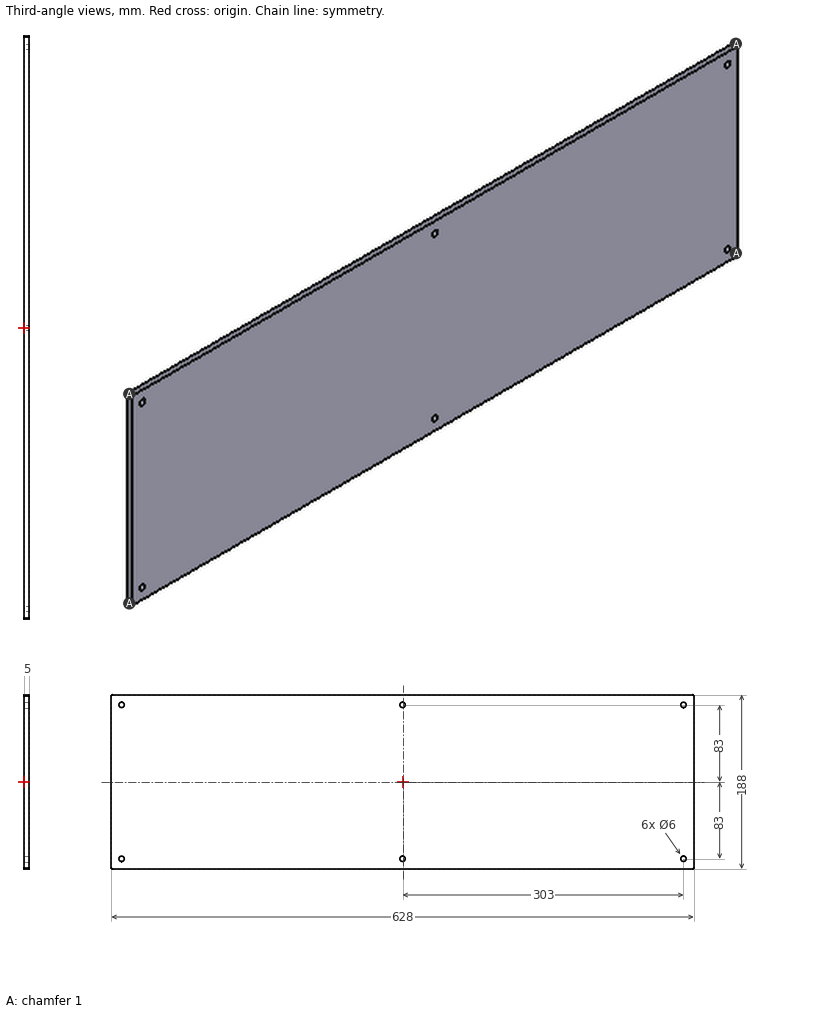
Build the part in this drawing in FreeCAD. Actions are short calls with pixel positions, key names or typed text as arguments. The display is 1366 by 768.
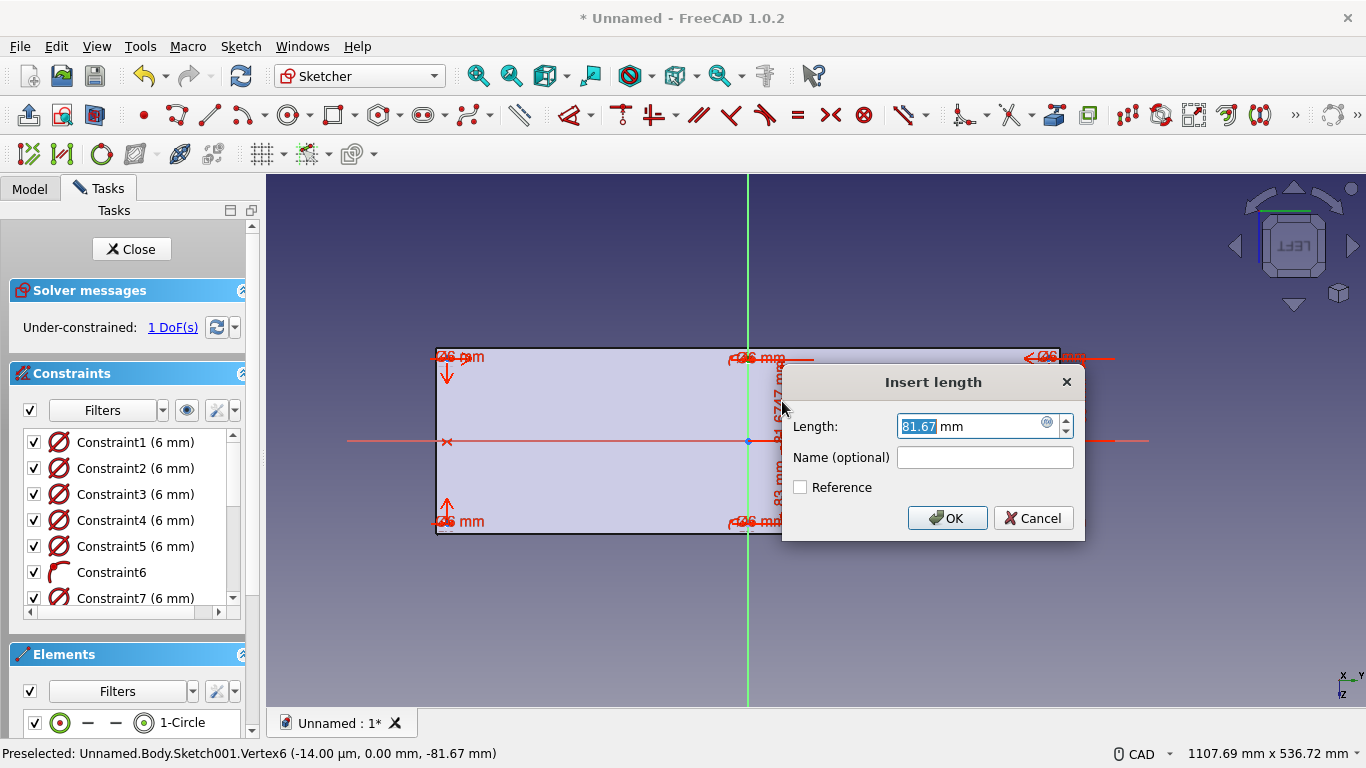
text(83)
key(Return)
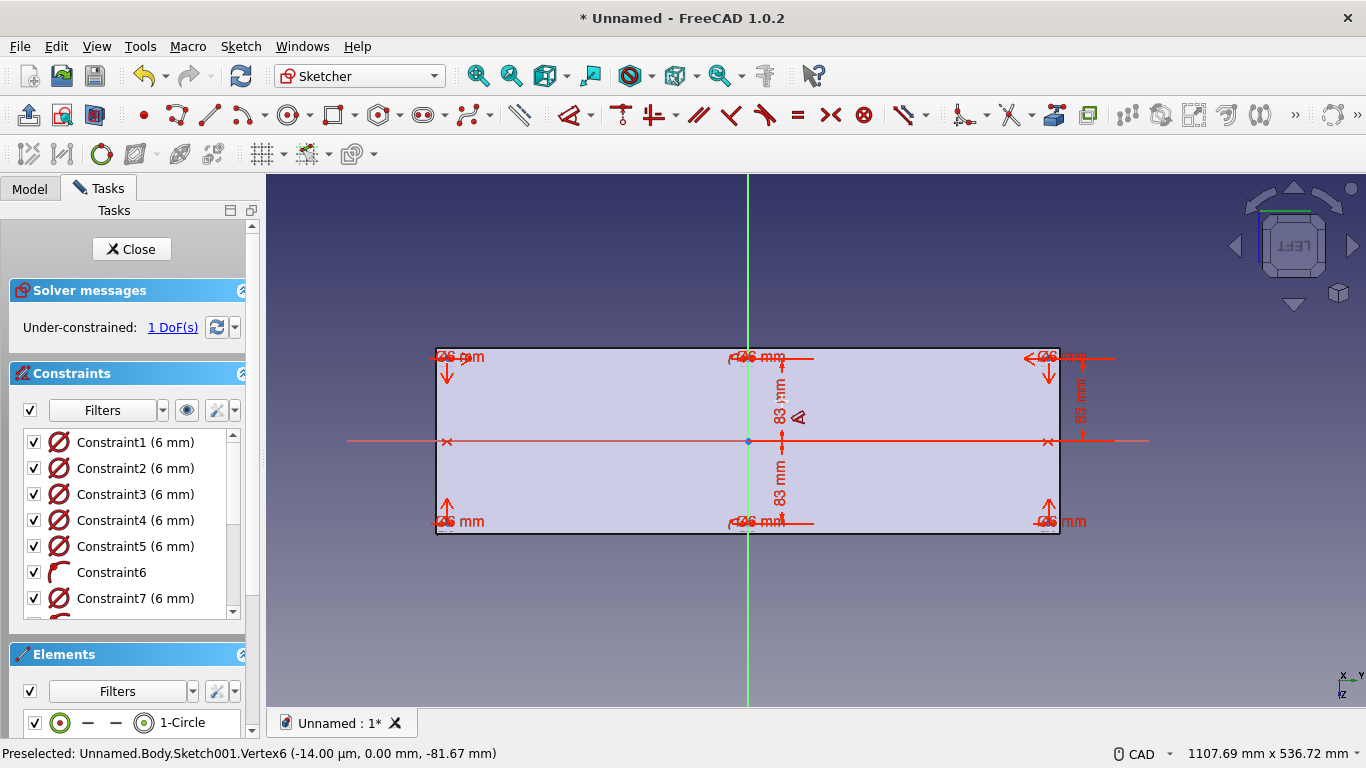
click(1049, 359)
click(899, 325)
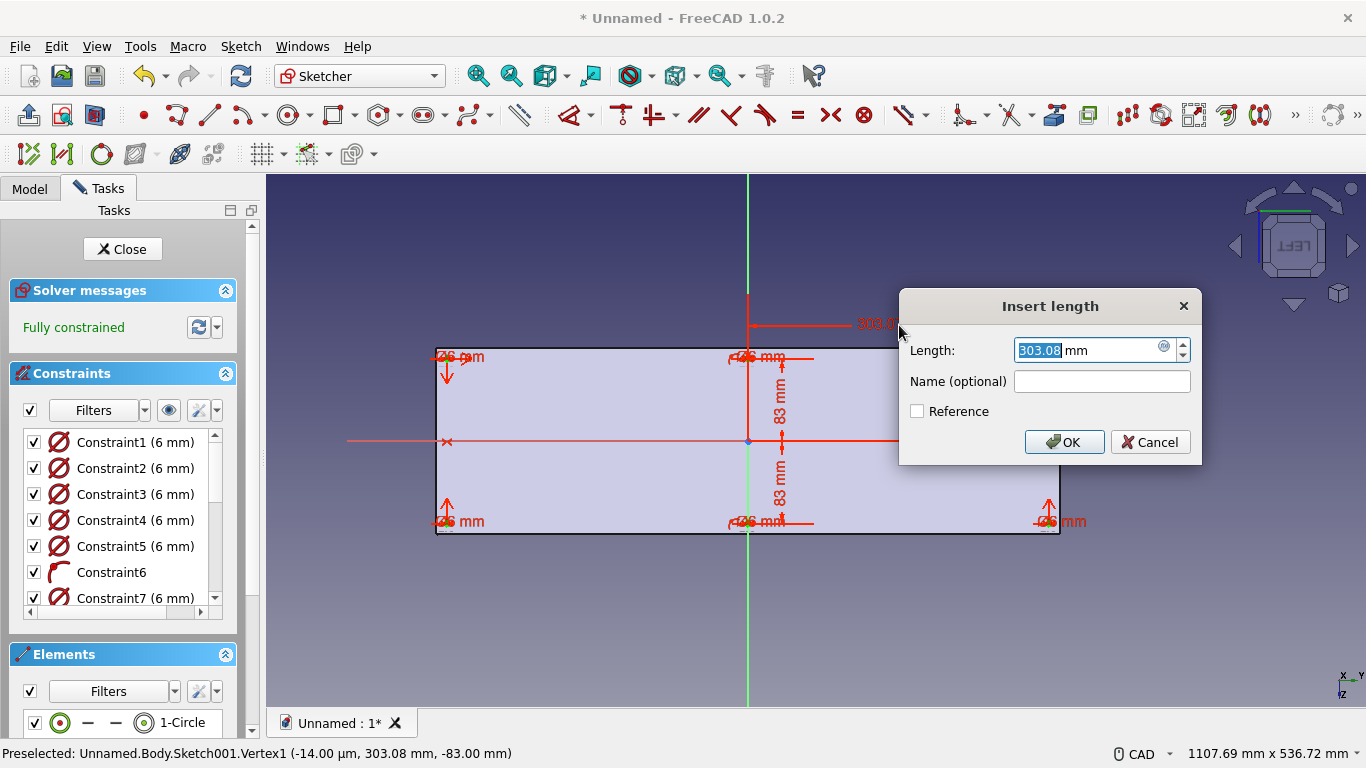
text(303)
key(Return)
key(Escape)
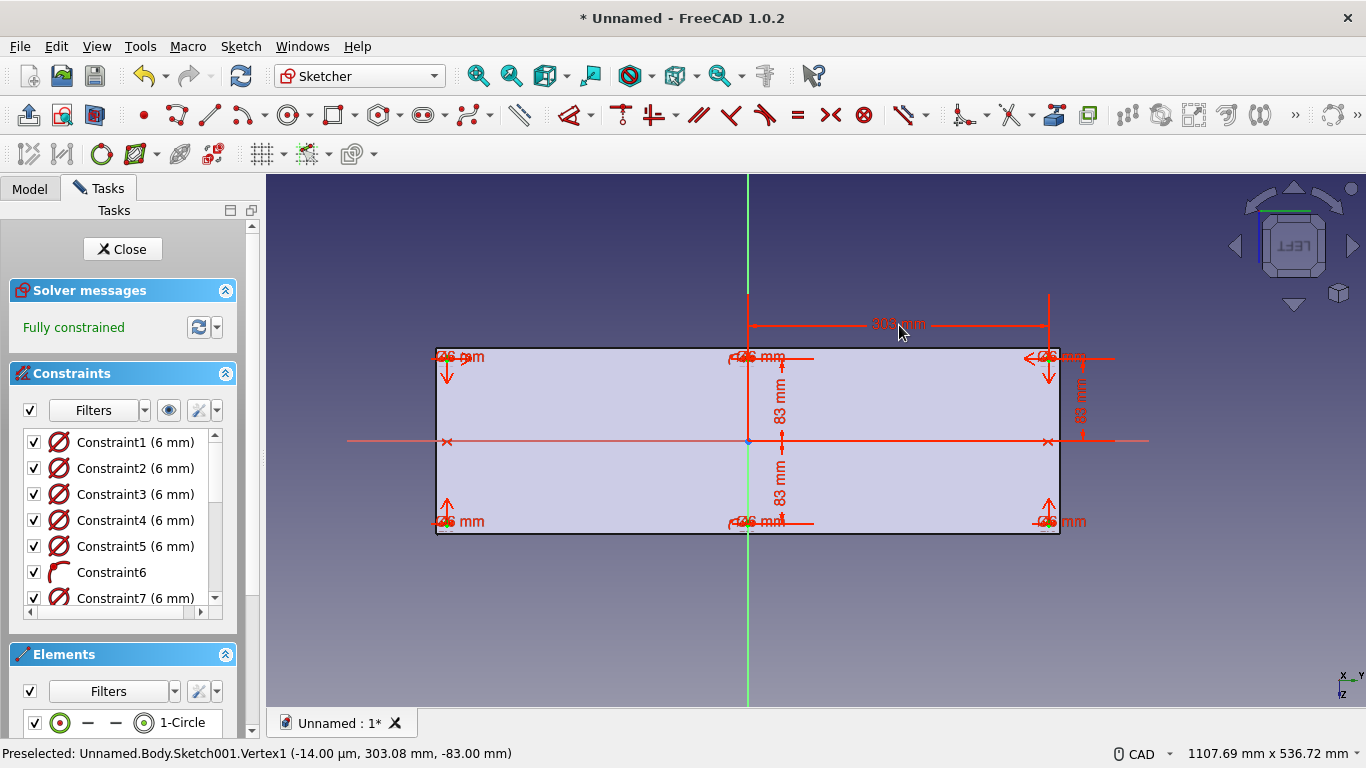
click(123, 249)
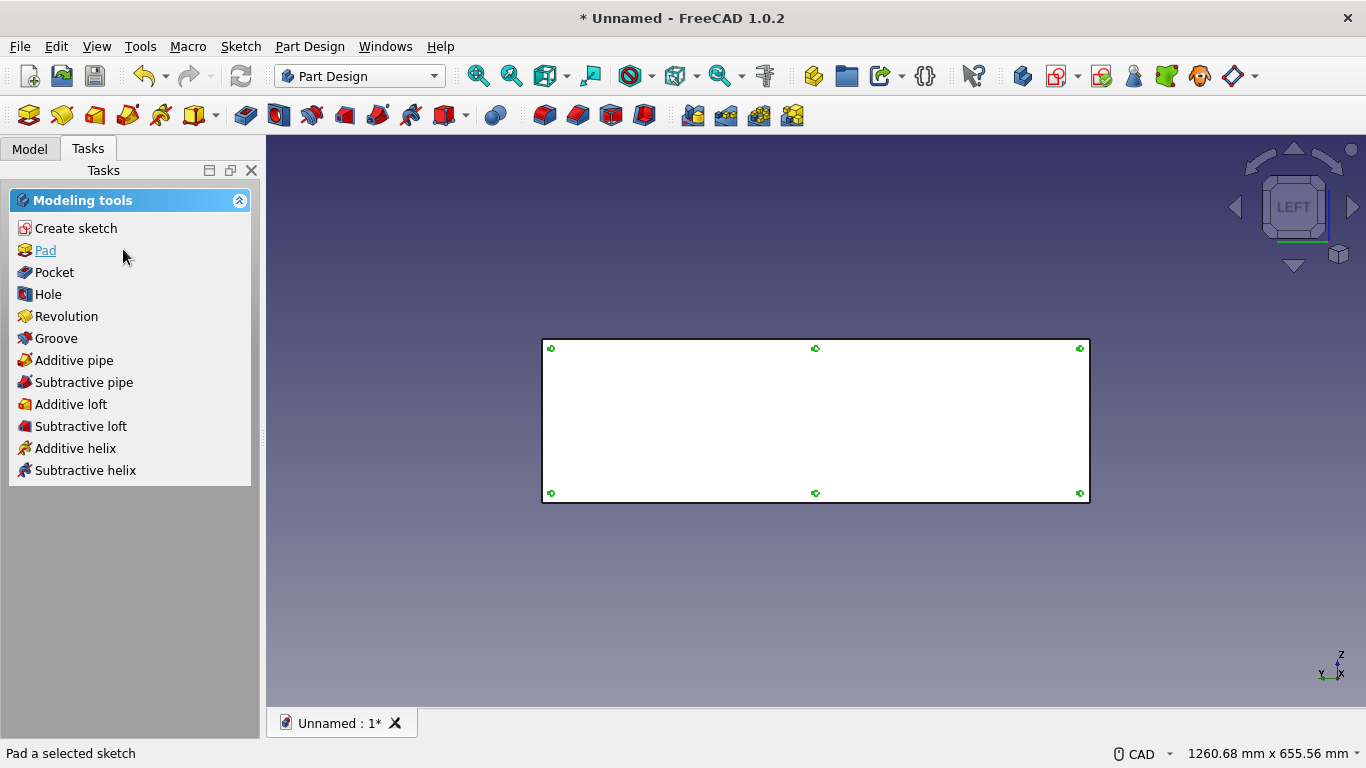
click(246, 116)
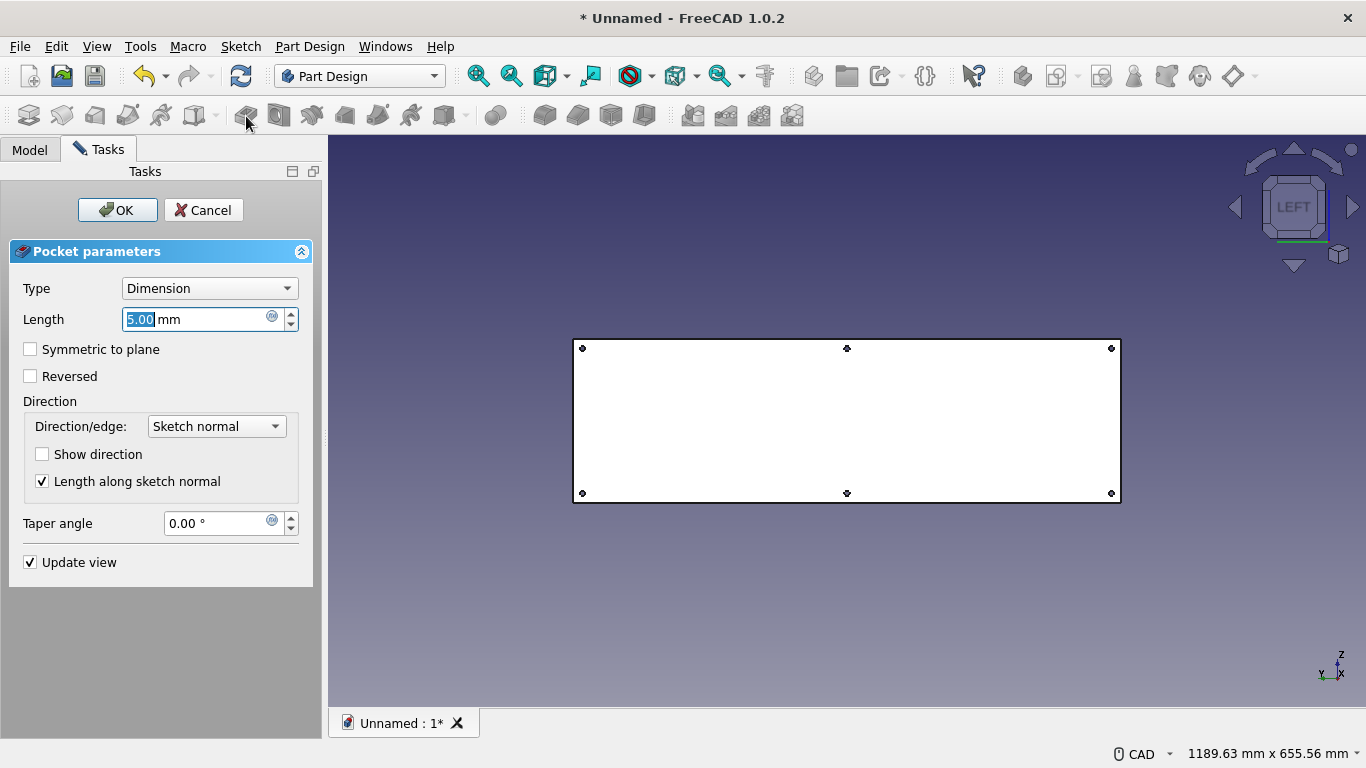
click(210, 288)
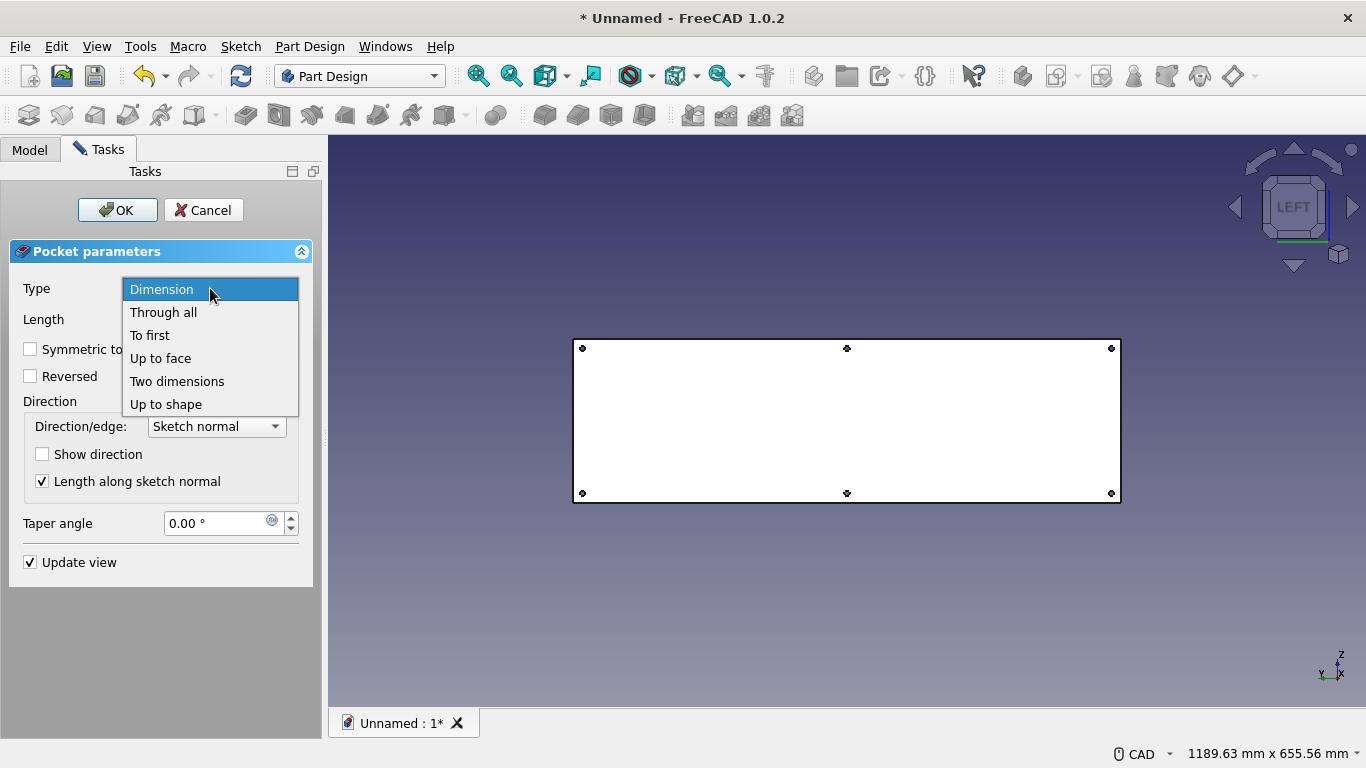
click(208, 312)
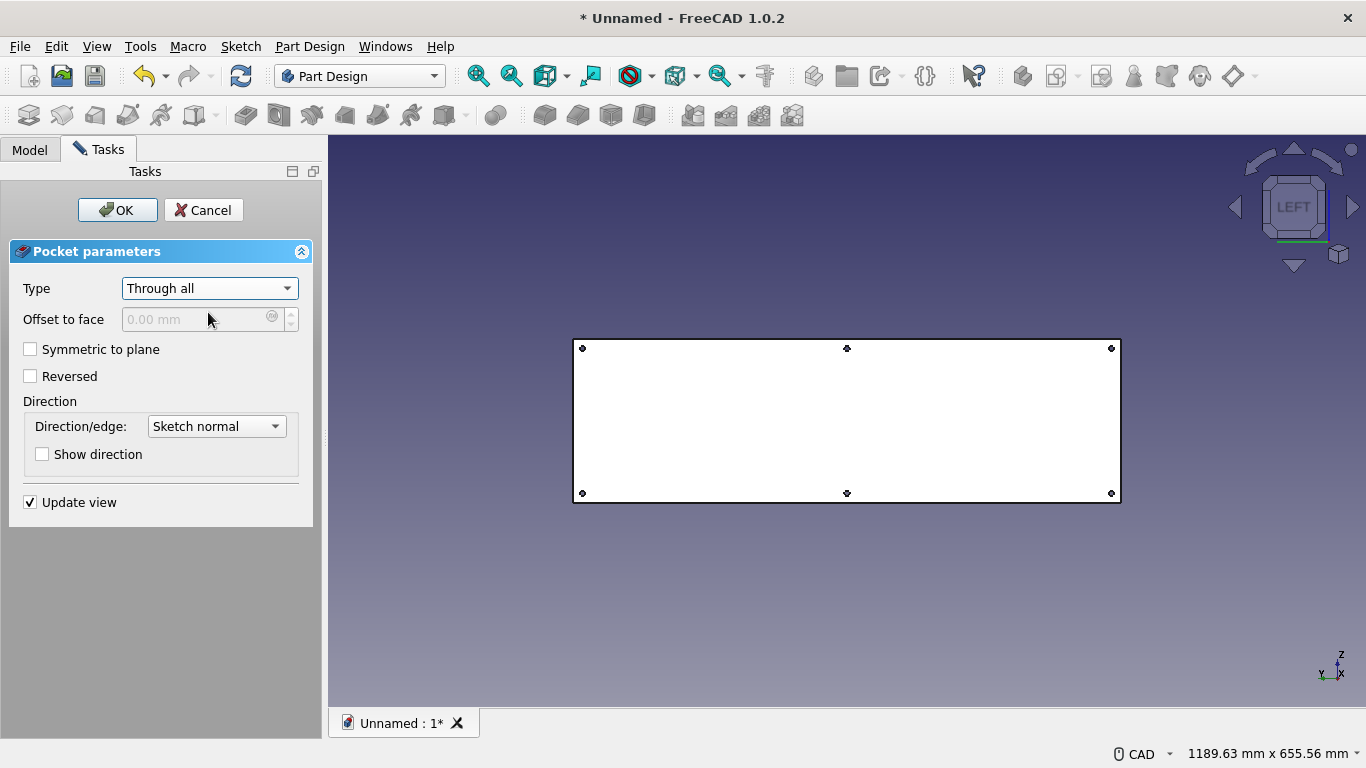
click(118, 210)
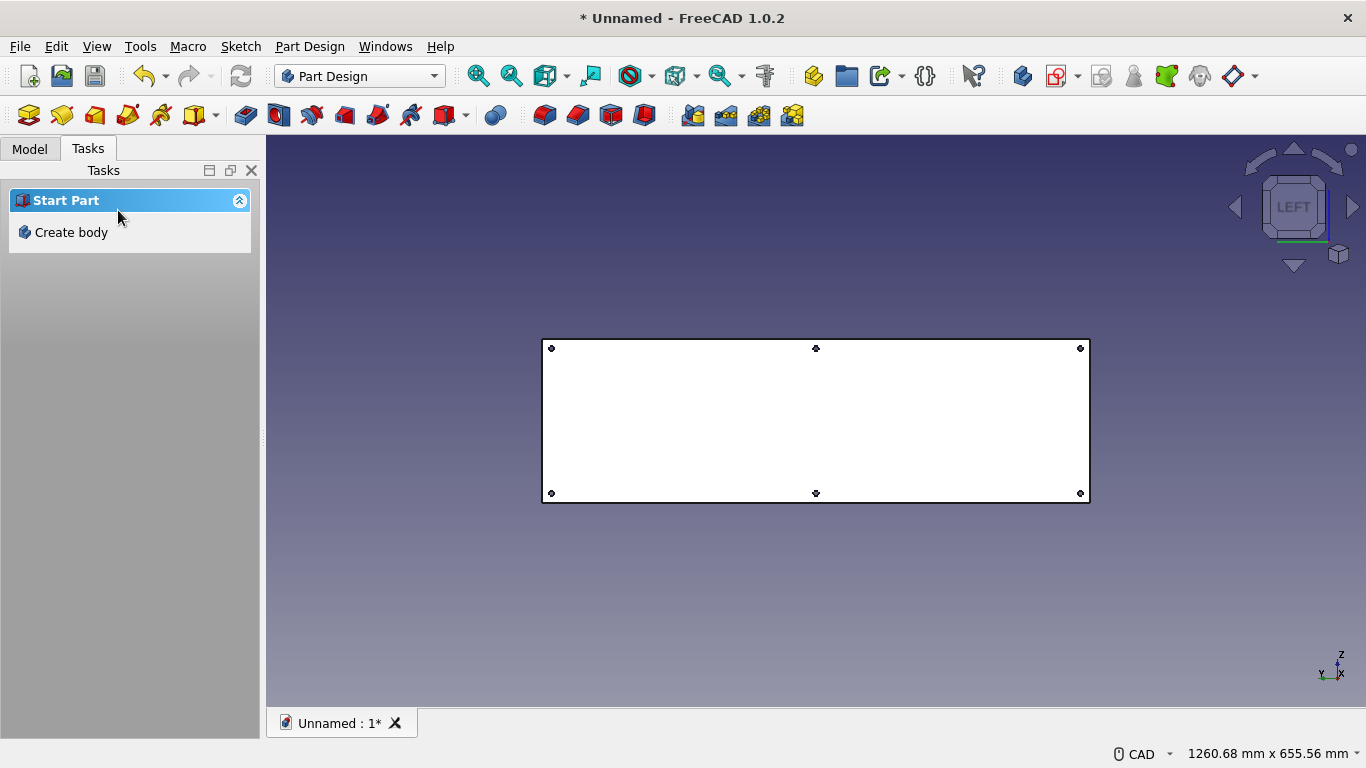
key(0)